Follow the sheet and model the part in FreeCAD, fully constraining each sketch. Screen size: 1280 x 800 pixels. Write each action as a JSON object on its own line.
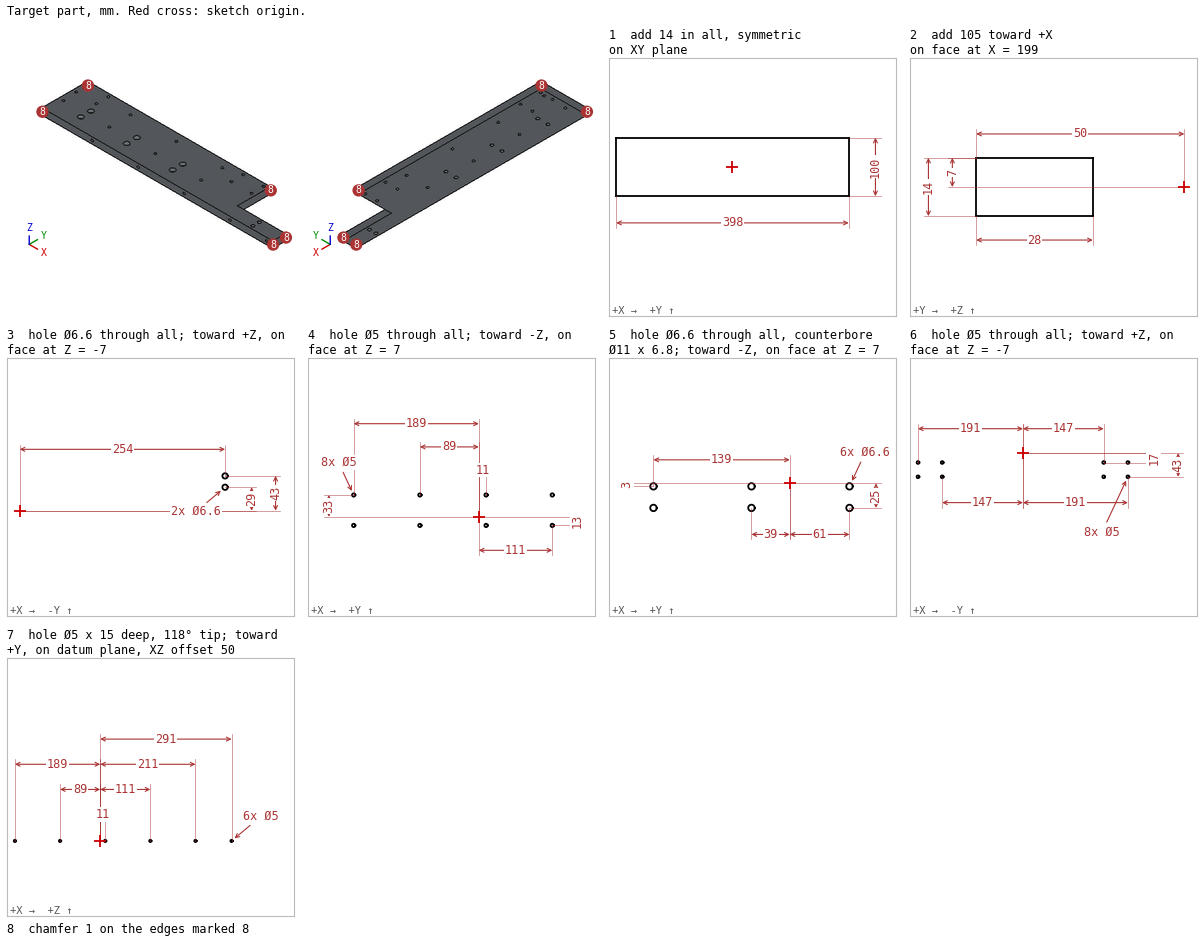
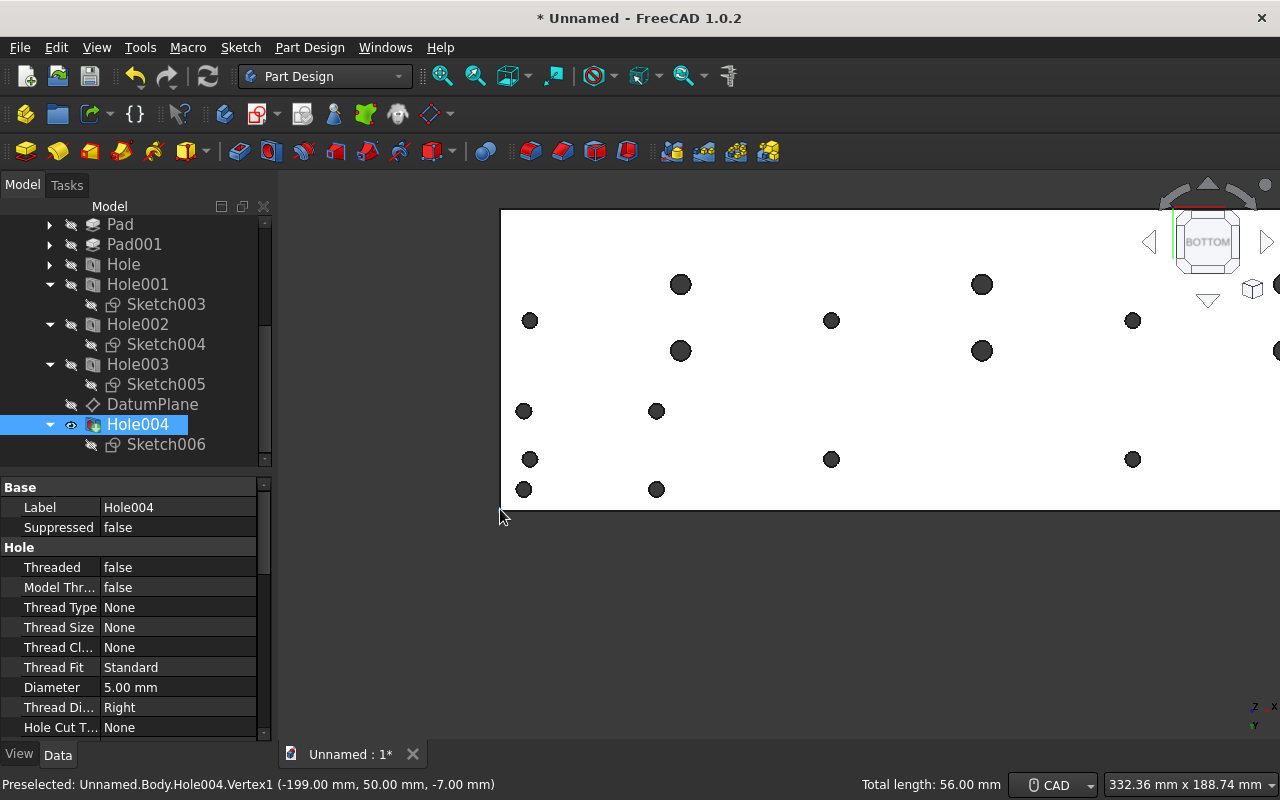
{"action": "key", "text": "v f"}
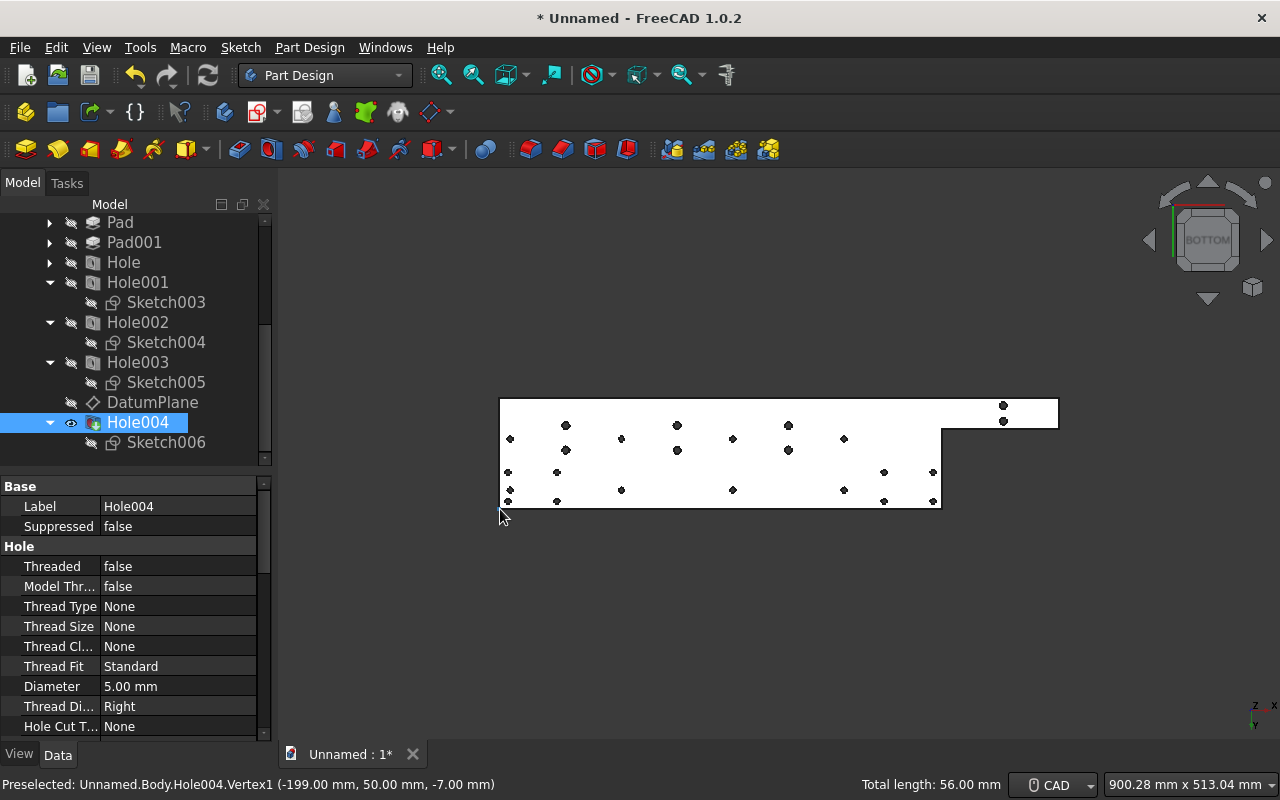
{"action": "key", "text": "4"}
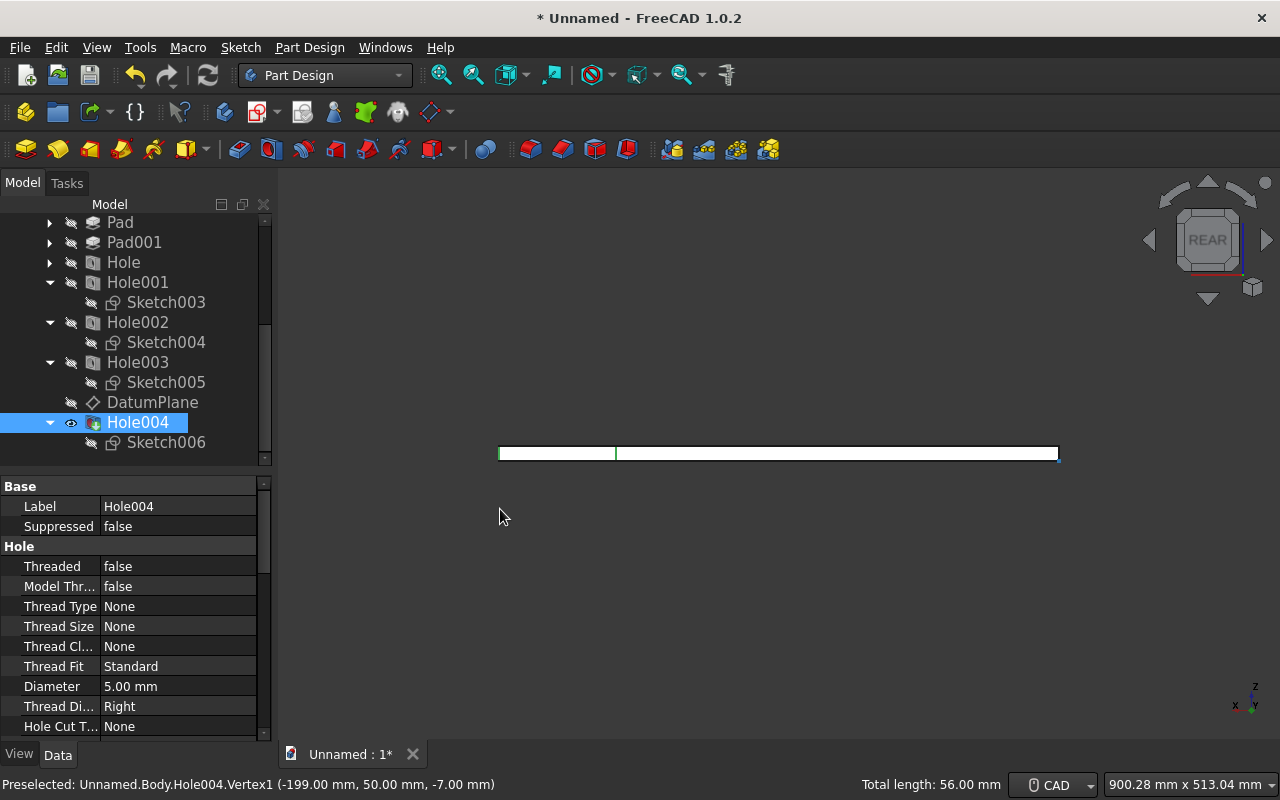
{"action": "left_click", "coordinate": [1059, 452], "text": "ctrl"}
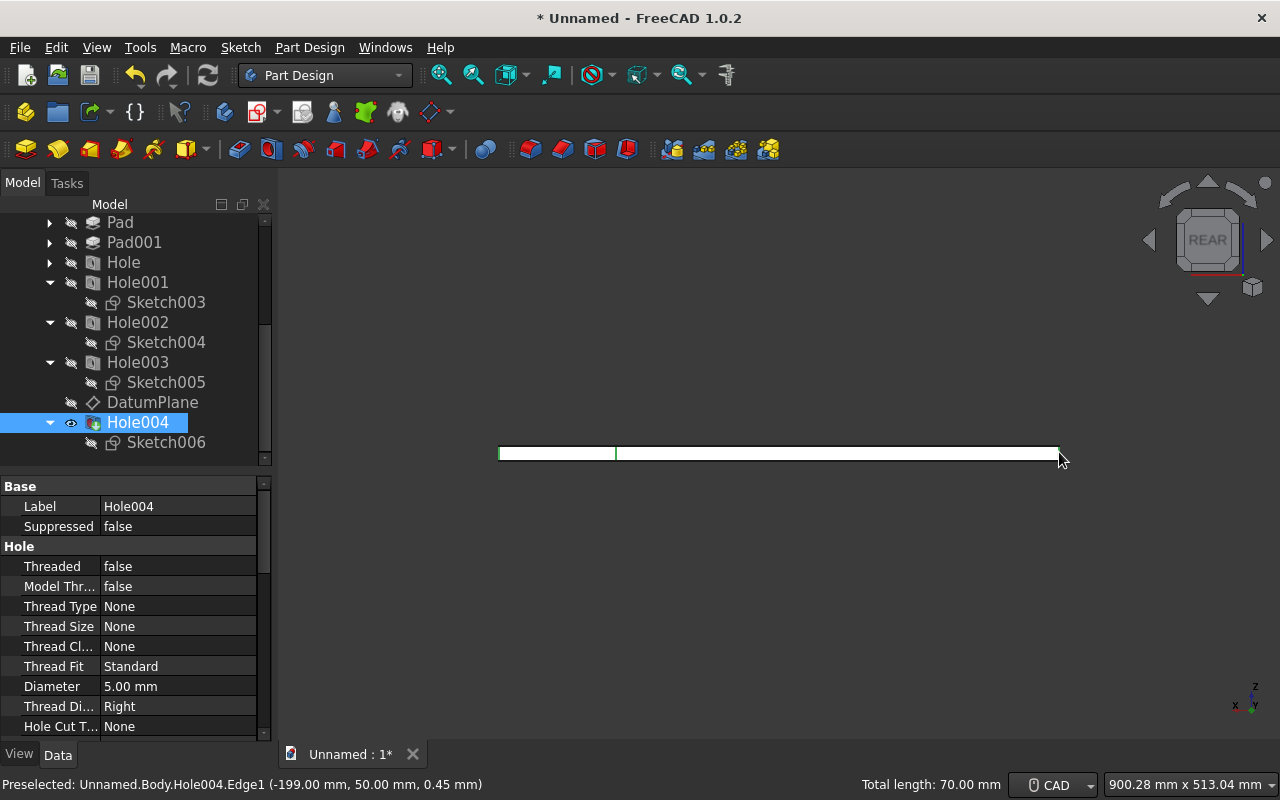
{"action": "left_click", "coordinate": [564, 150]}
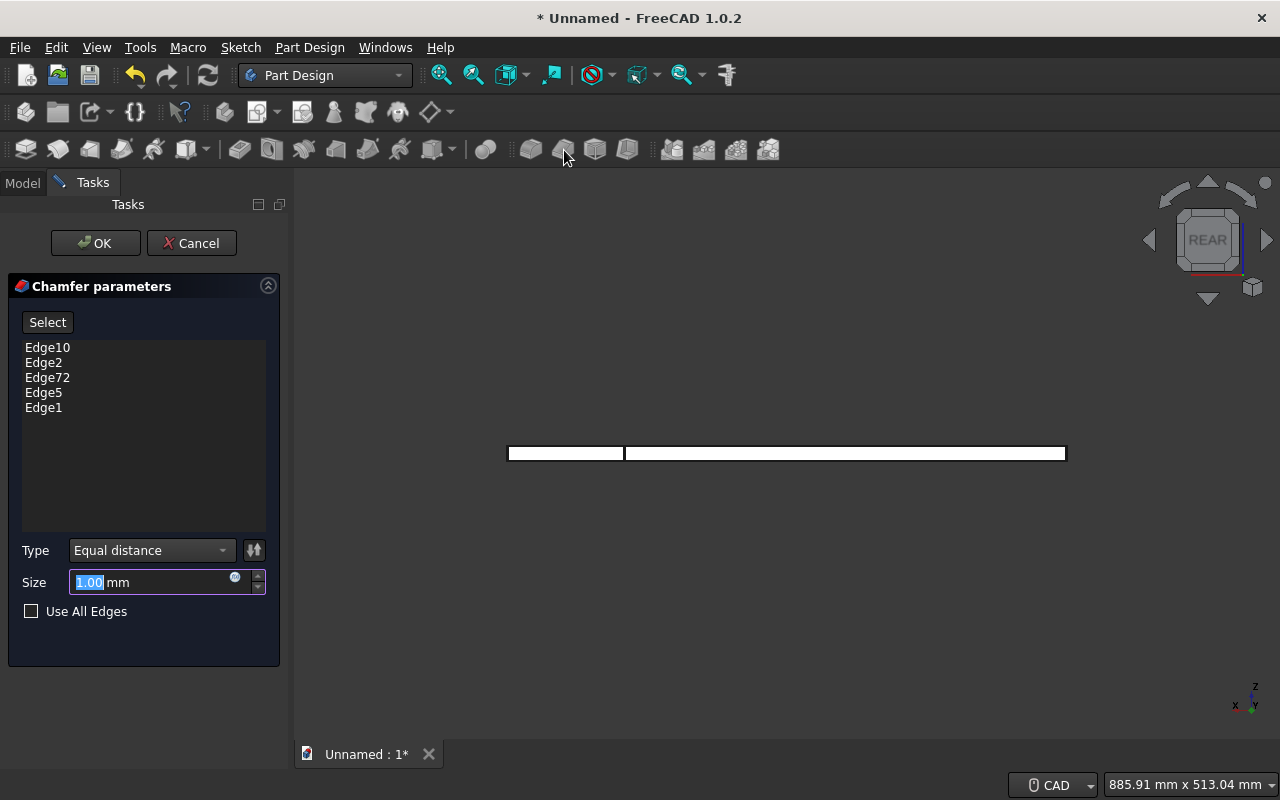
{"action": "type", "text": "1"}
{"action": "key", "text": "Tab"}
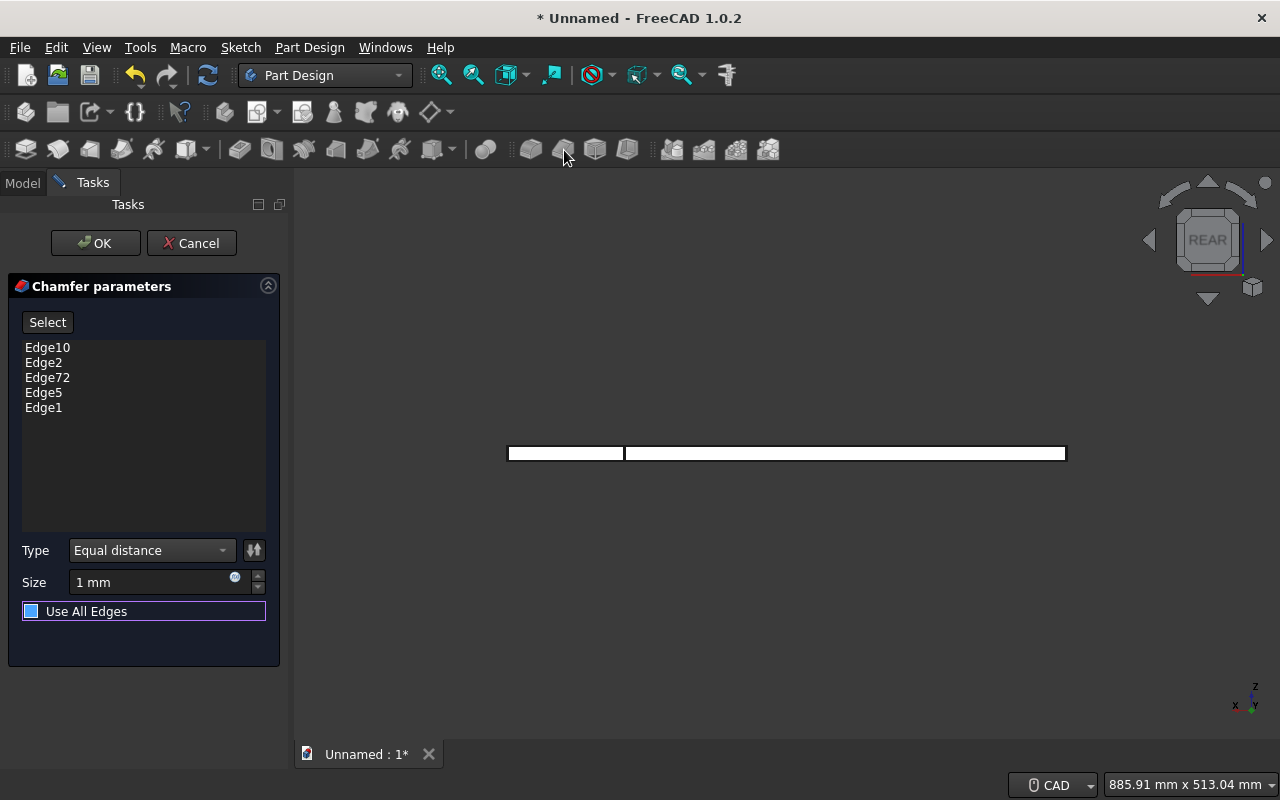
{"action": "left_click", "coordinate": [96, 243]}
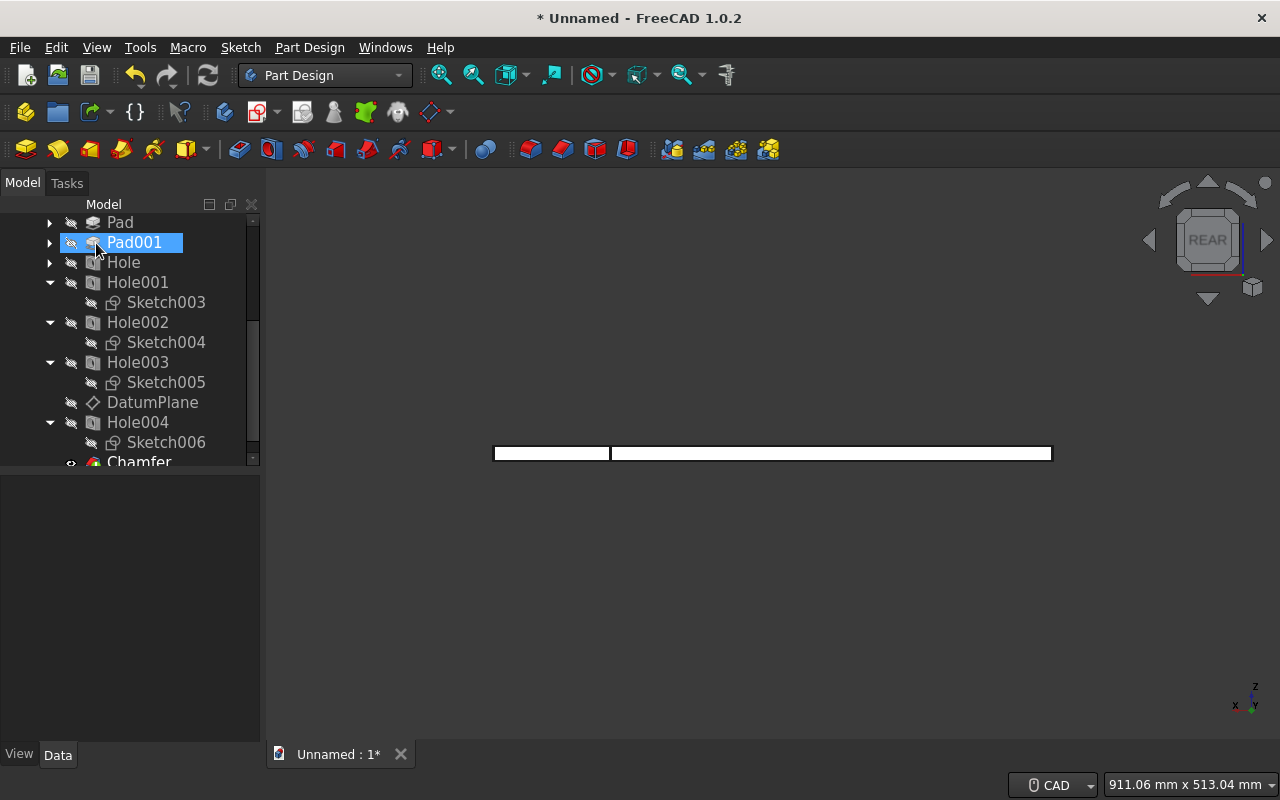
{"action": "key", "text": "0"}